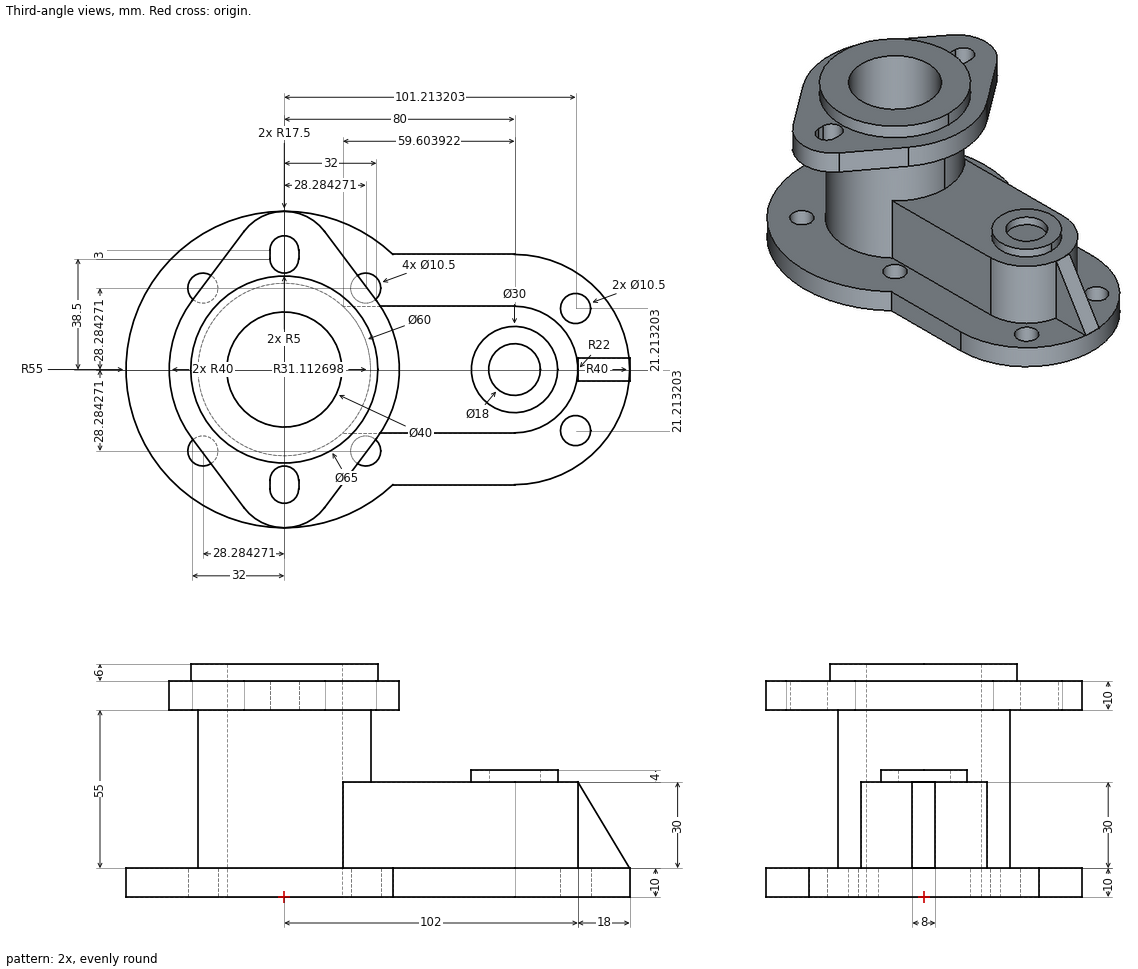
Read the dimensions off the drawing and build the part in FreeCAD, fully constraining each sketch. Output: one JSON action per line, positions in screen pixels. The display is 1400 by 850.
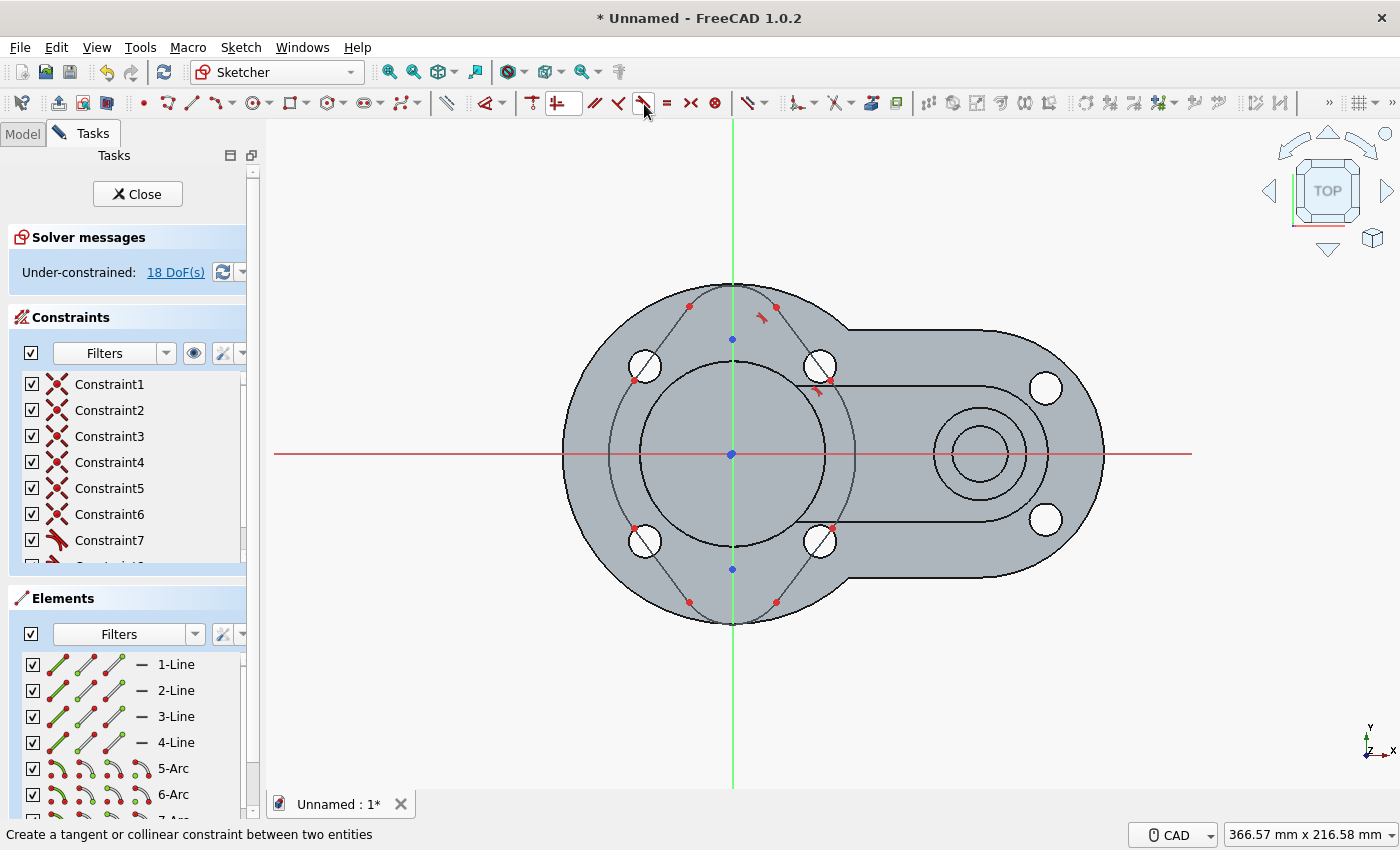
{"action": "left_click", "coordinate": [673, 329]}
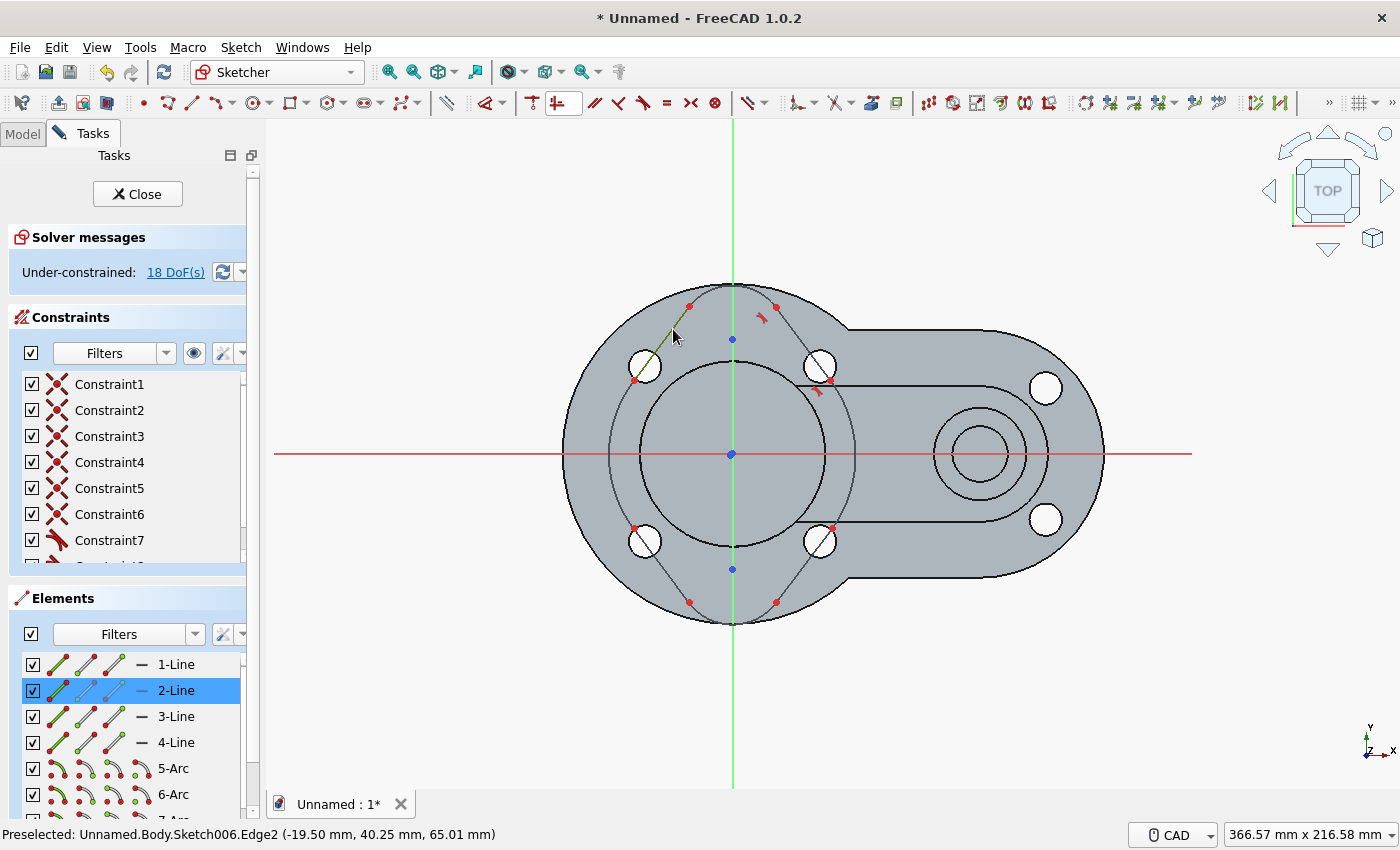
{"action": "left_click", "coordinate": [752, 289]}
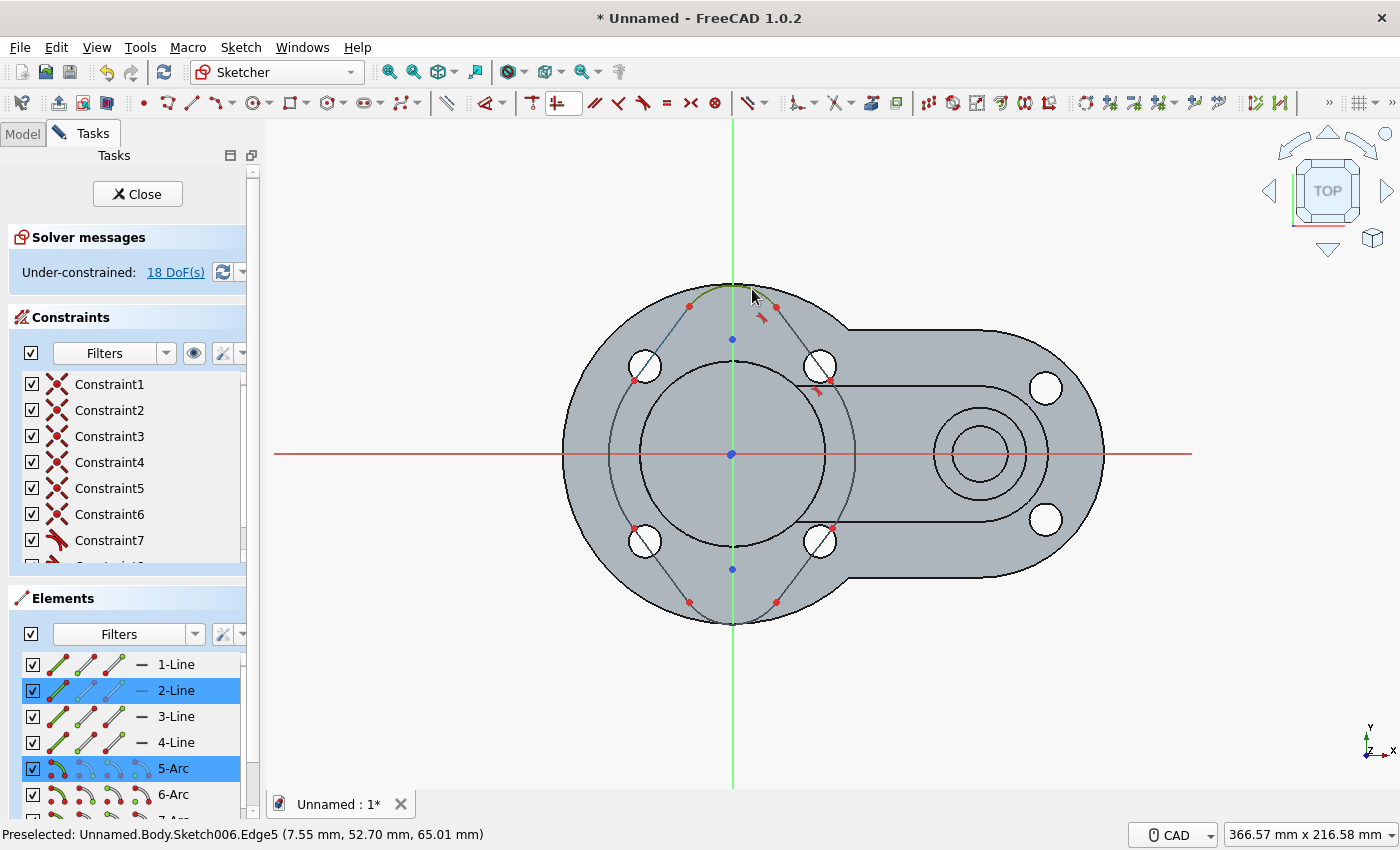
{"action": "key", "text": "t"}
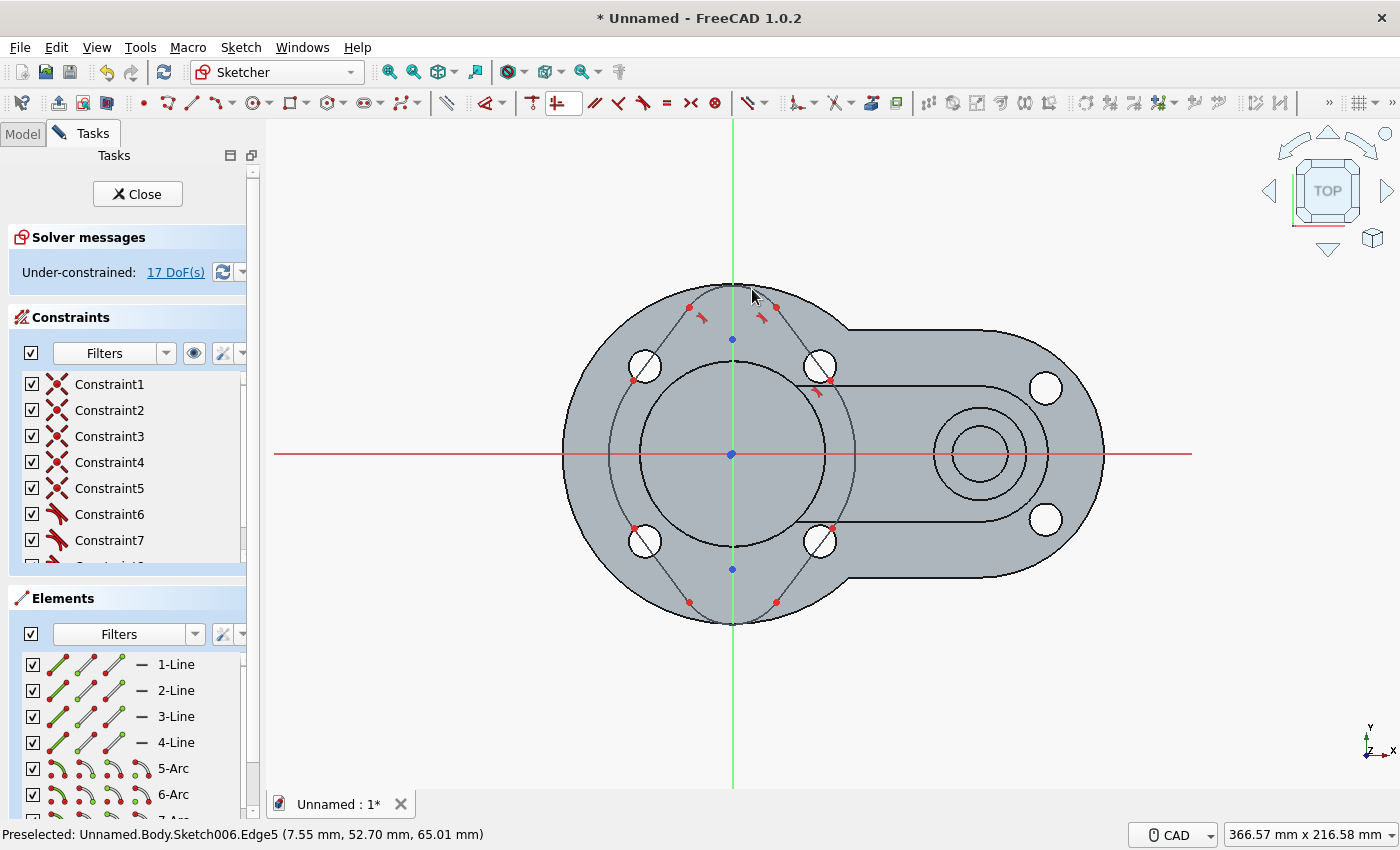
{"action": "left_click", "coordinate": [672, 330]}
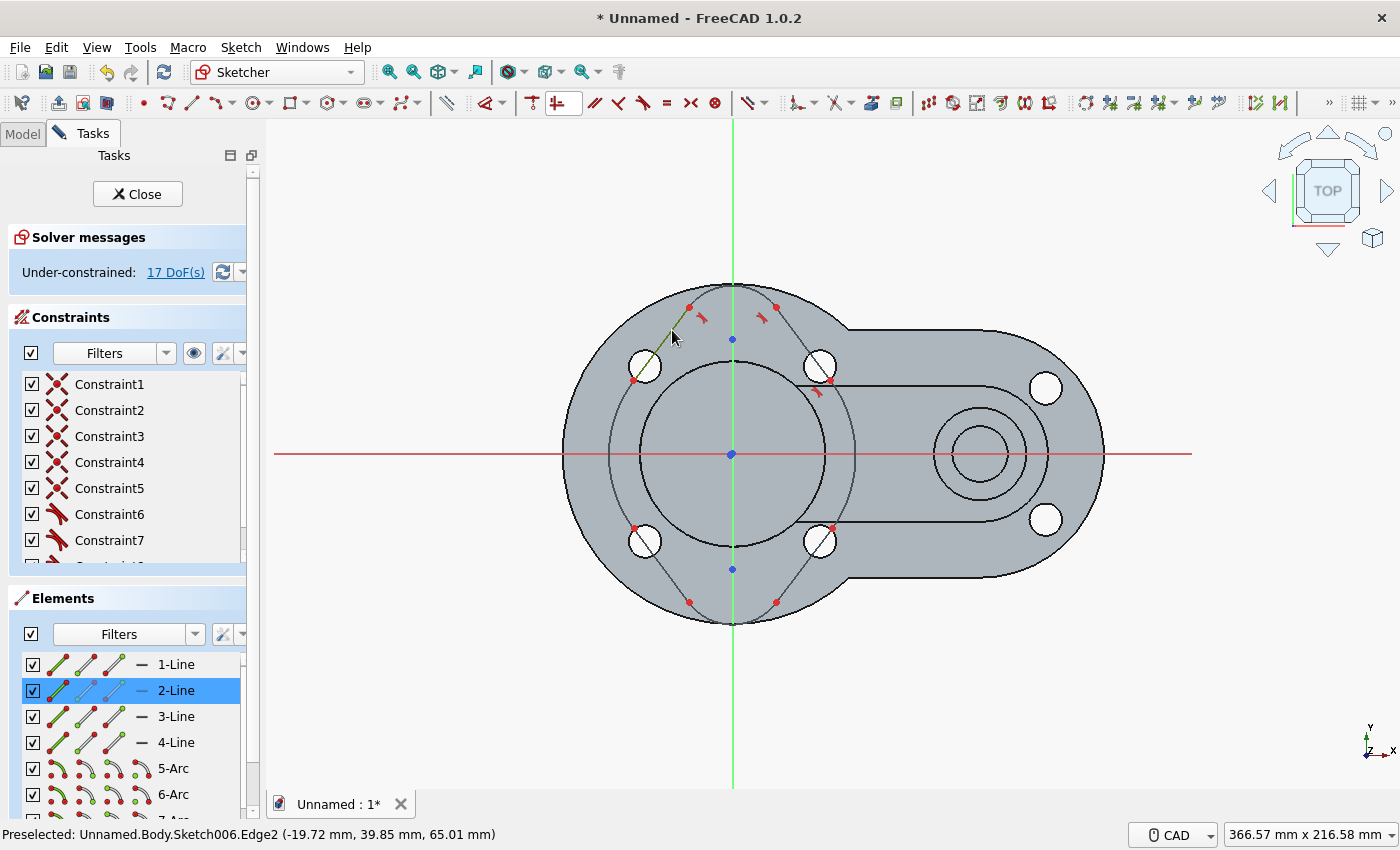
{"action": "left_click", "coordinate": [613, 424]}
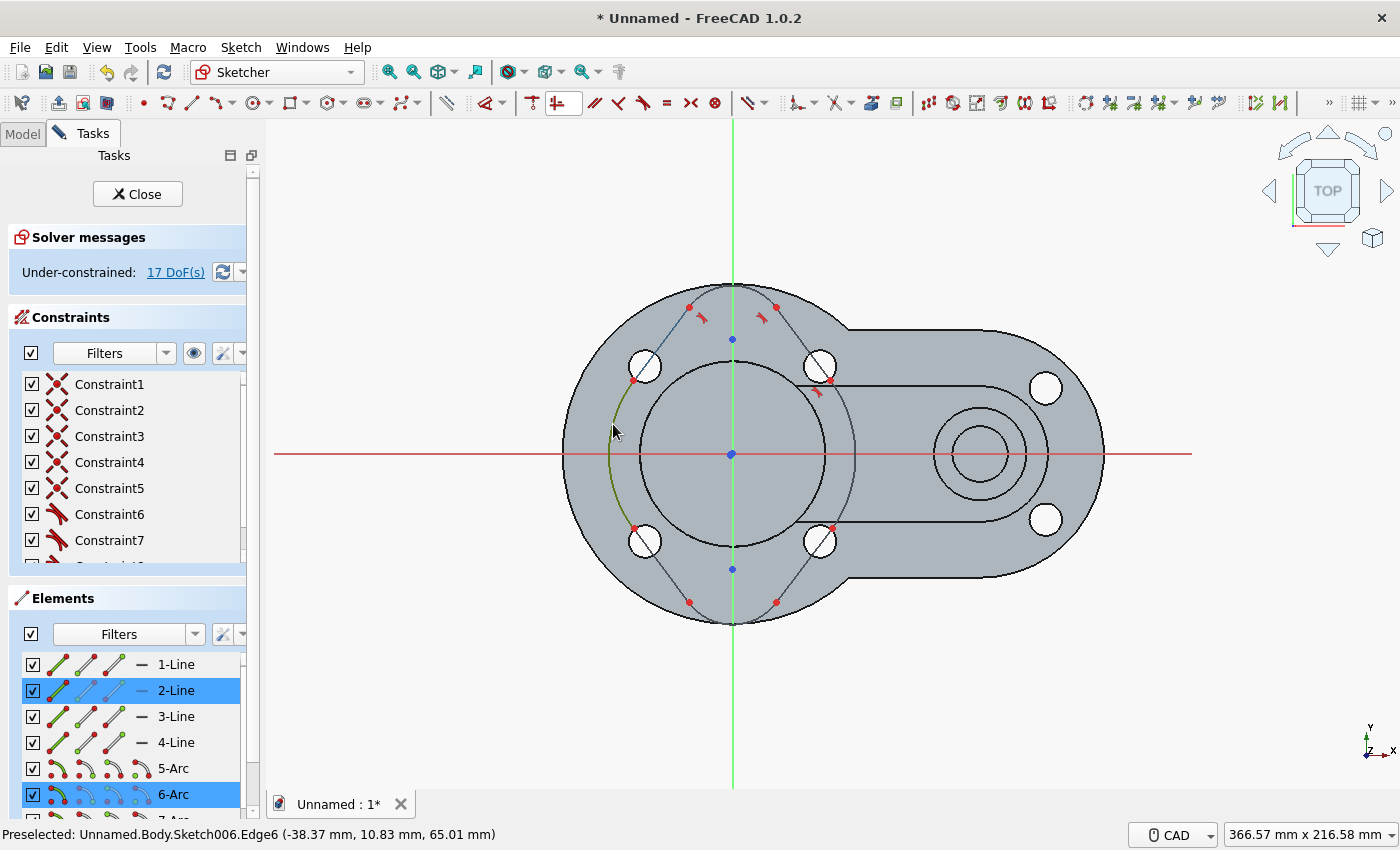
{"action": "key", "text": "t"}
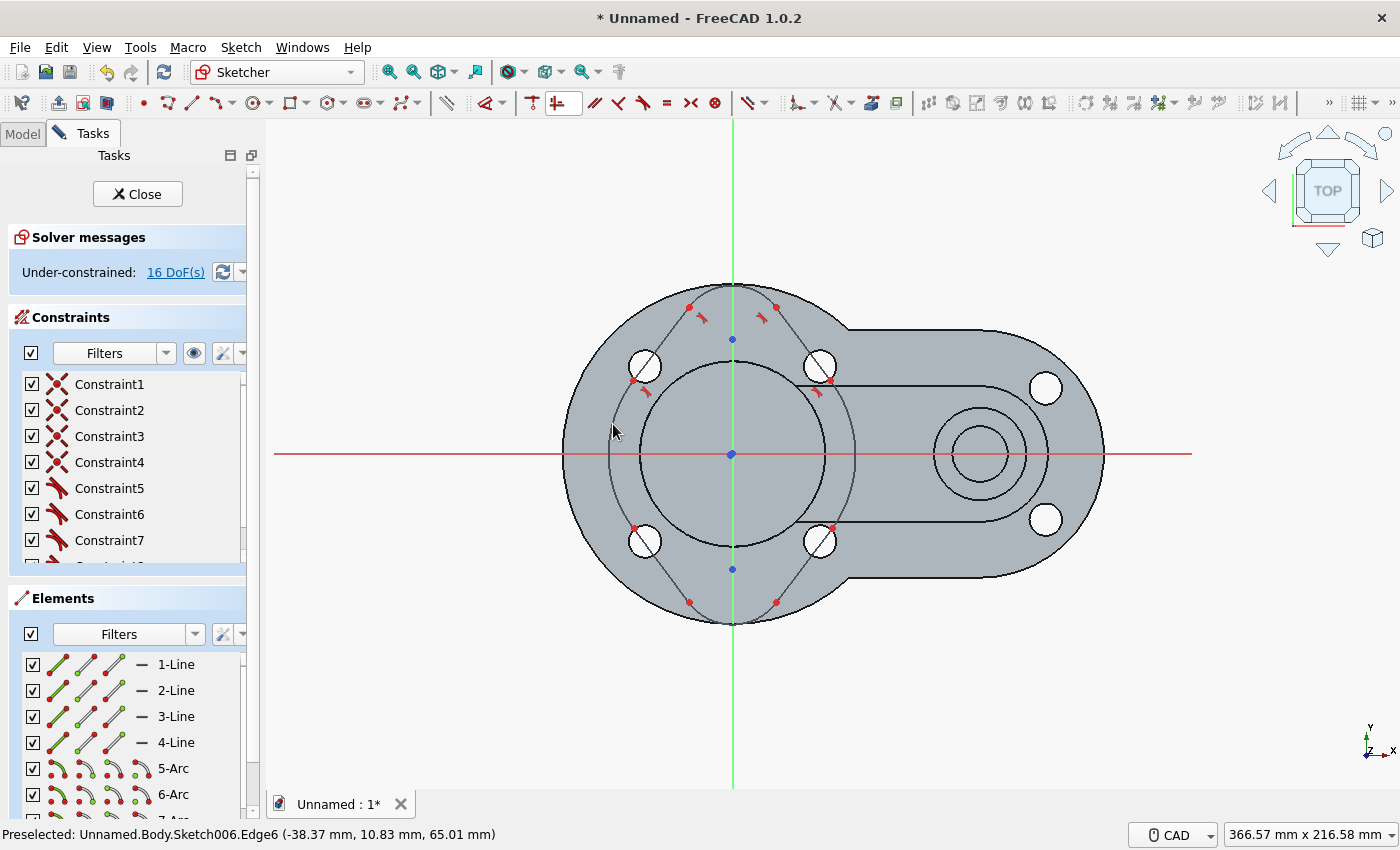
{"action": "left_click", "coordinate": [651, 551]}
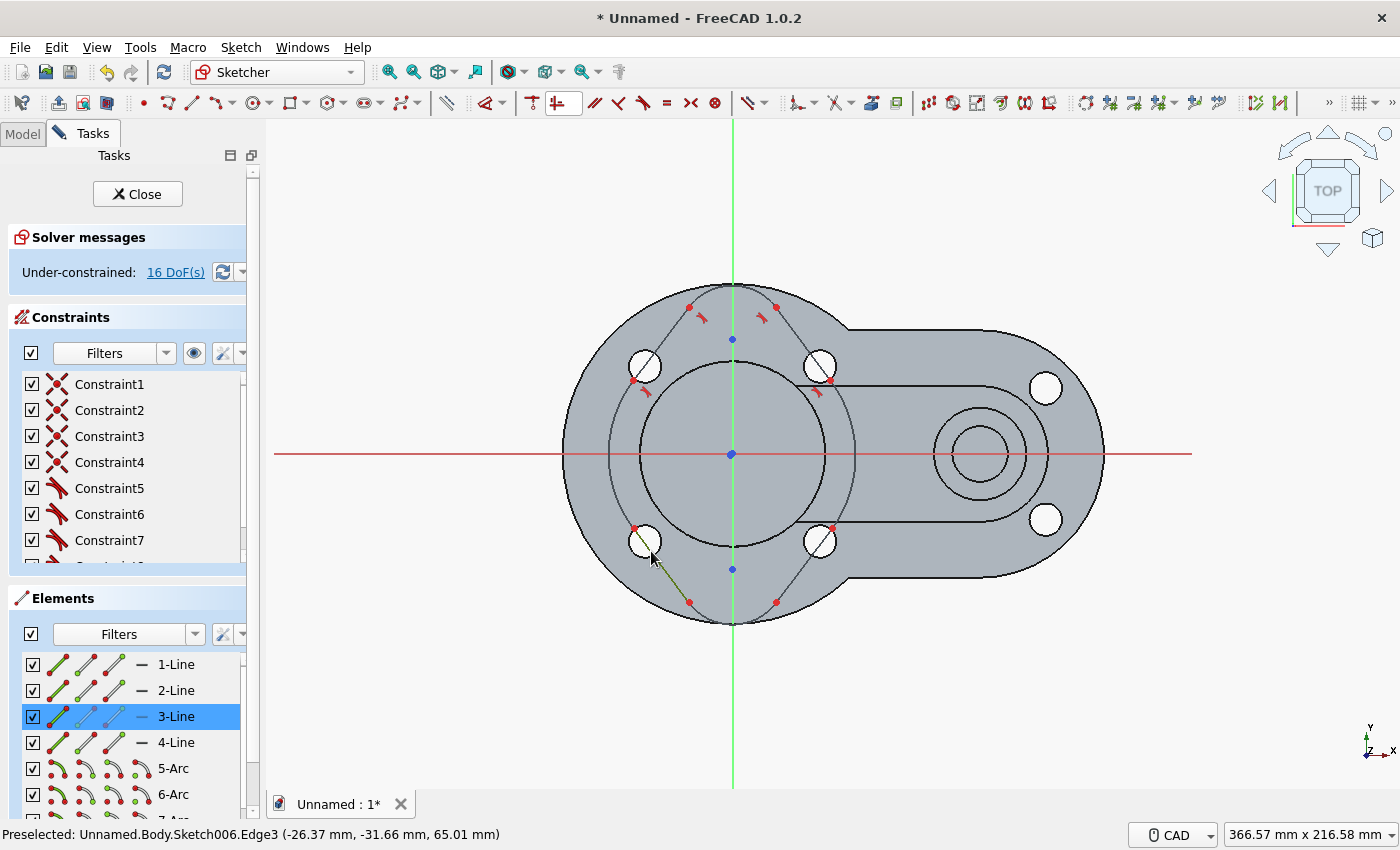
{"action": "left_click", "coordinate": [613, 424]}